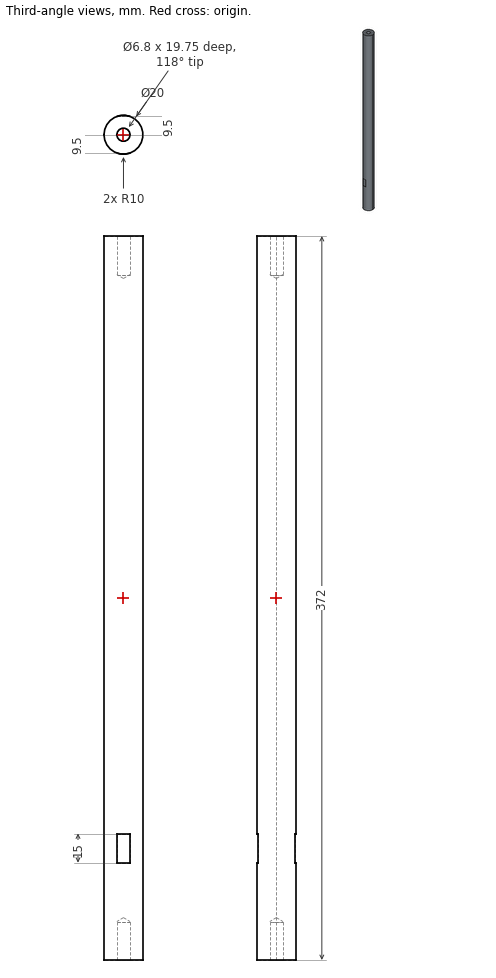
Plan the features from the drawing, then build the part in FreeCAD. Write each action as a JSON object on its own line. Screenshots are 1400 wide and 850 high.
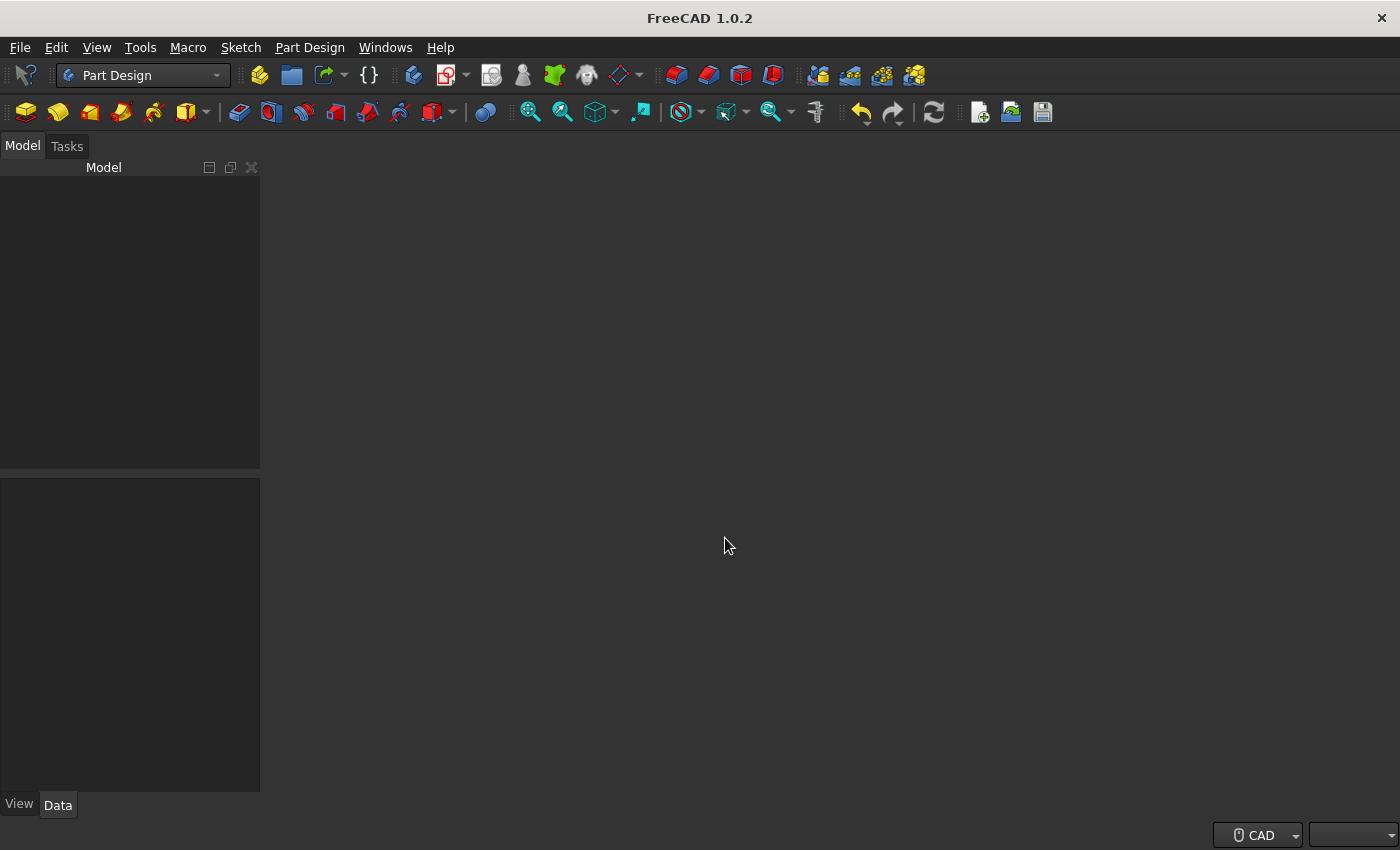
{"action": "left_click", "coordinate": [980, 112]}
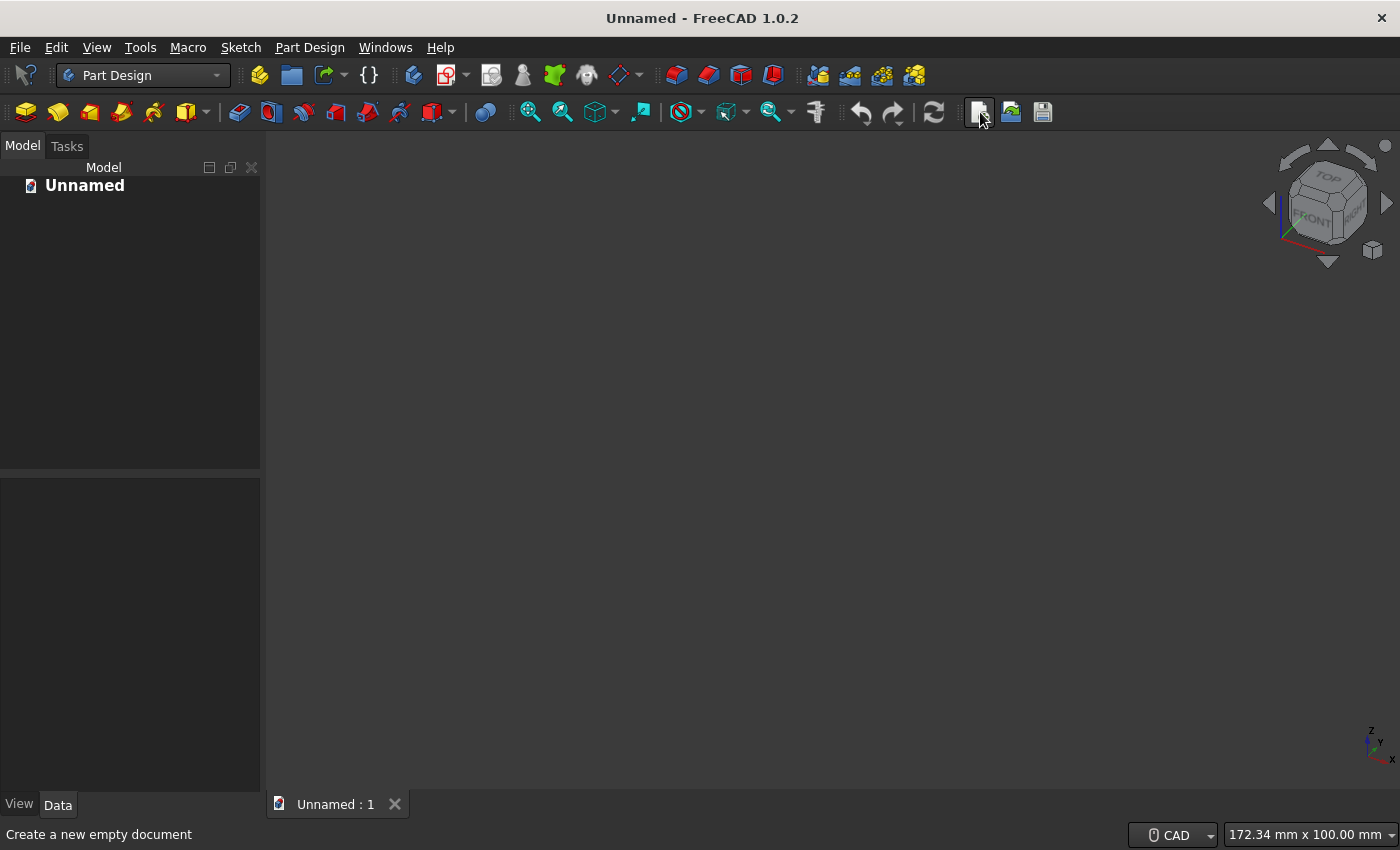
{"action": "left_click", "coordinate": [446, 76]}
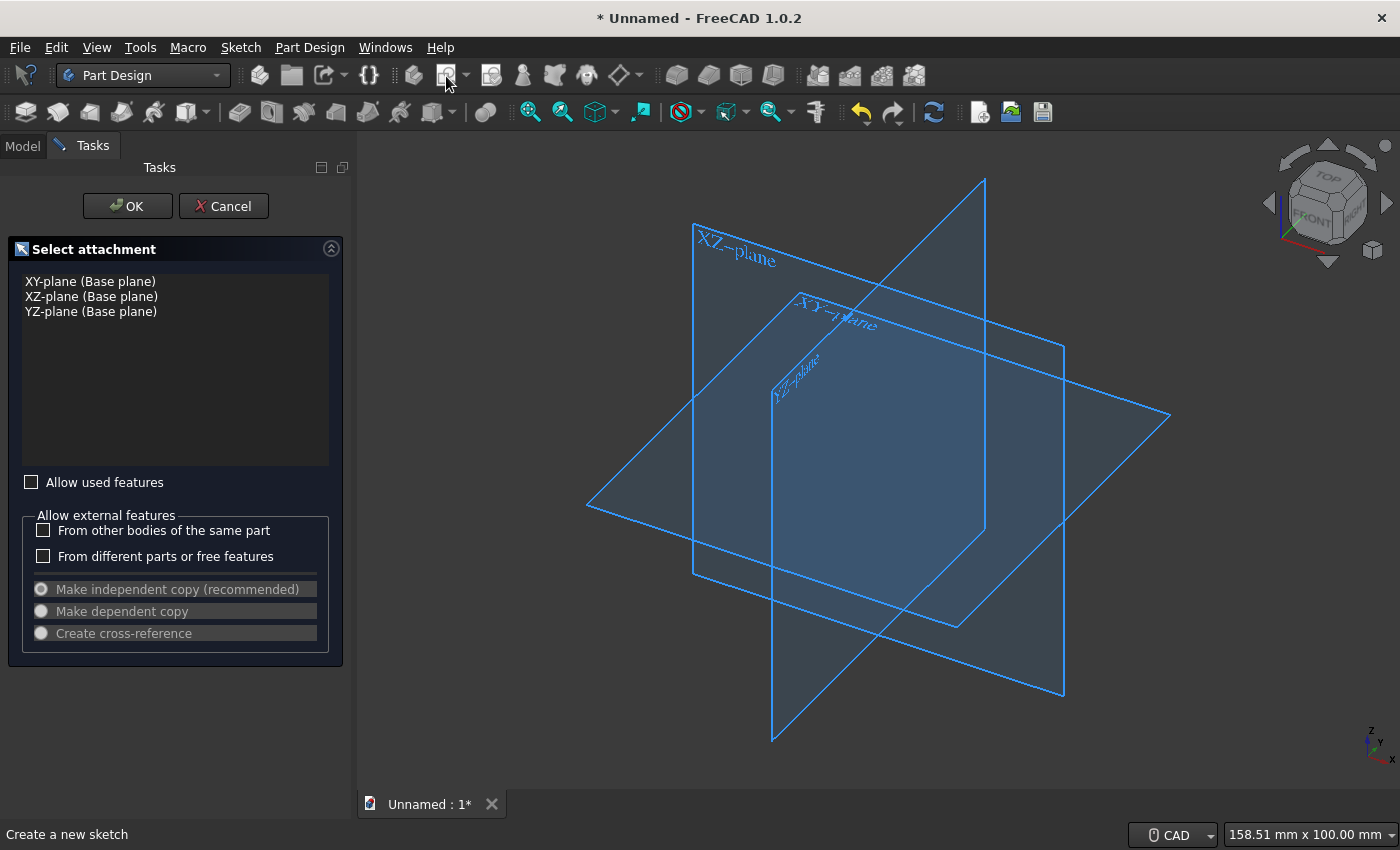
{"action": "left_click", "coordinate": [82, 282]}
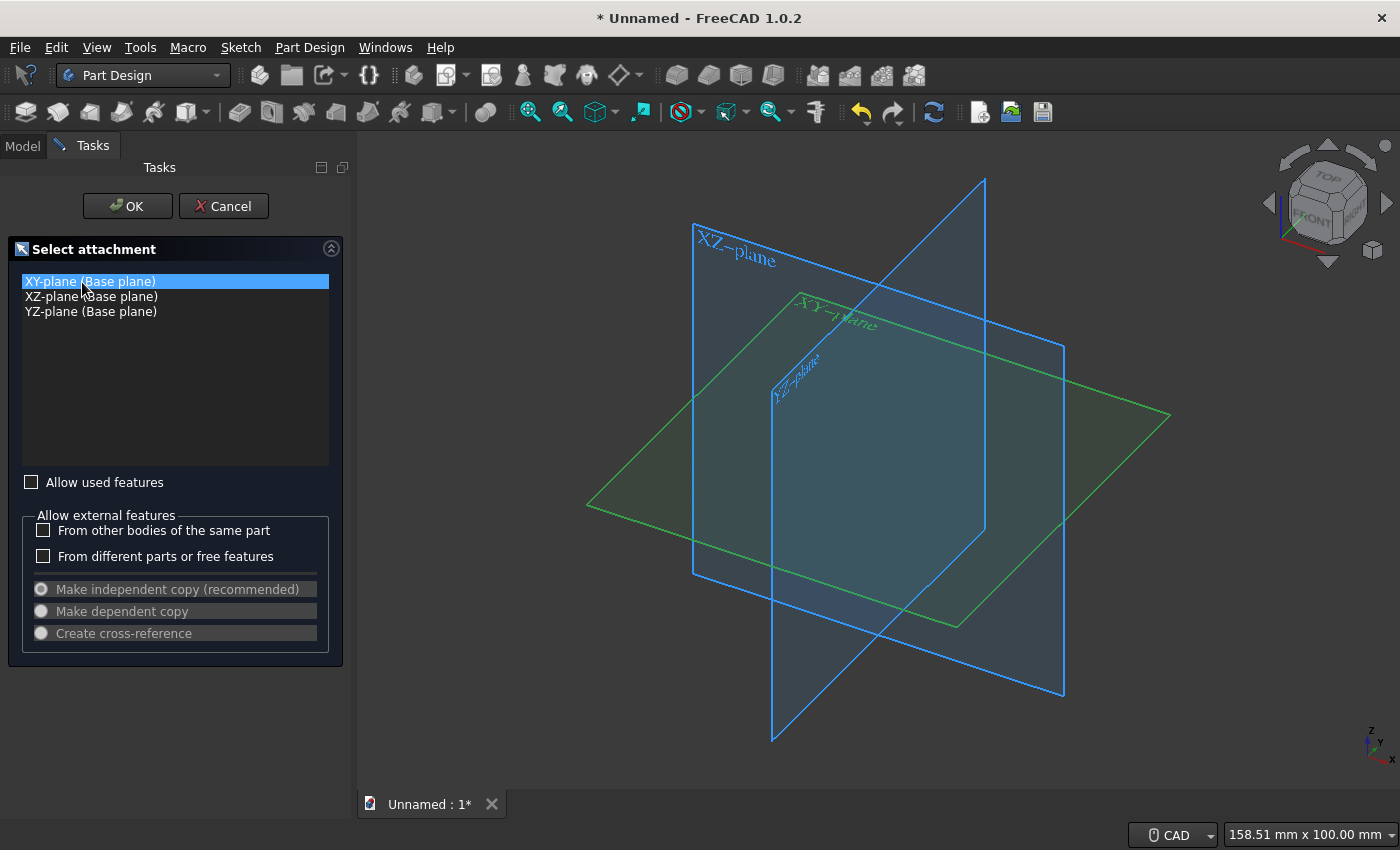
{"action": "left_click", "coordinate": [128, 206]}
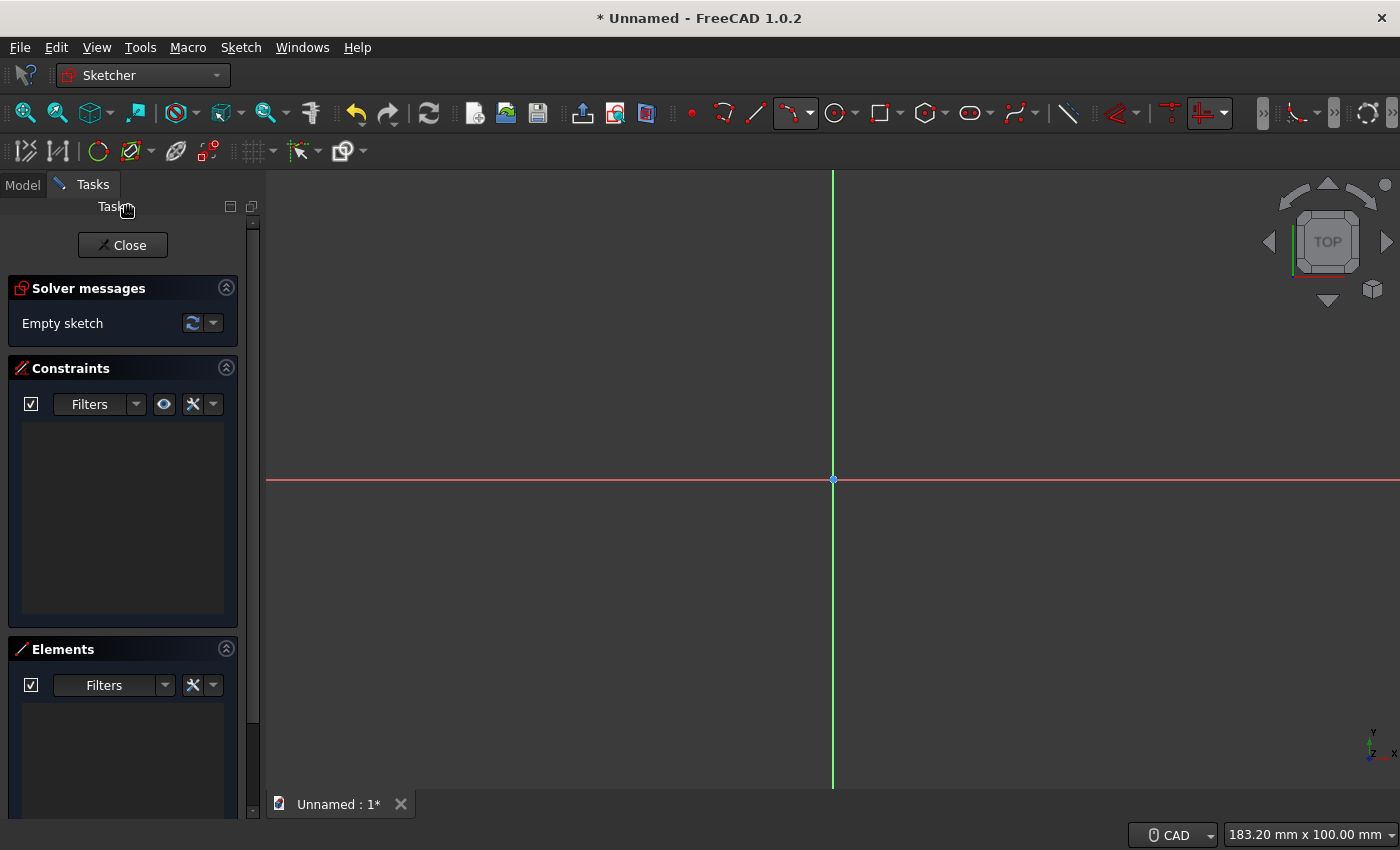
{"action": "scroll", "coordinate": [863, 480], "scroll_direction": "up", "scroll_amount": 6}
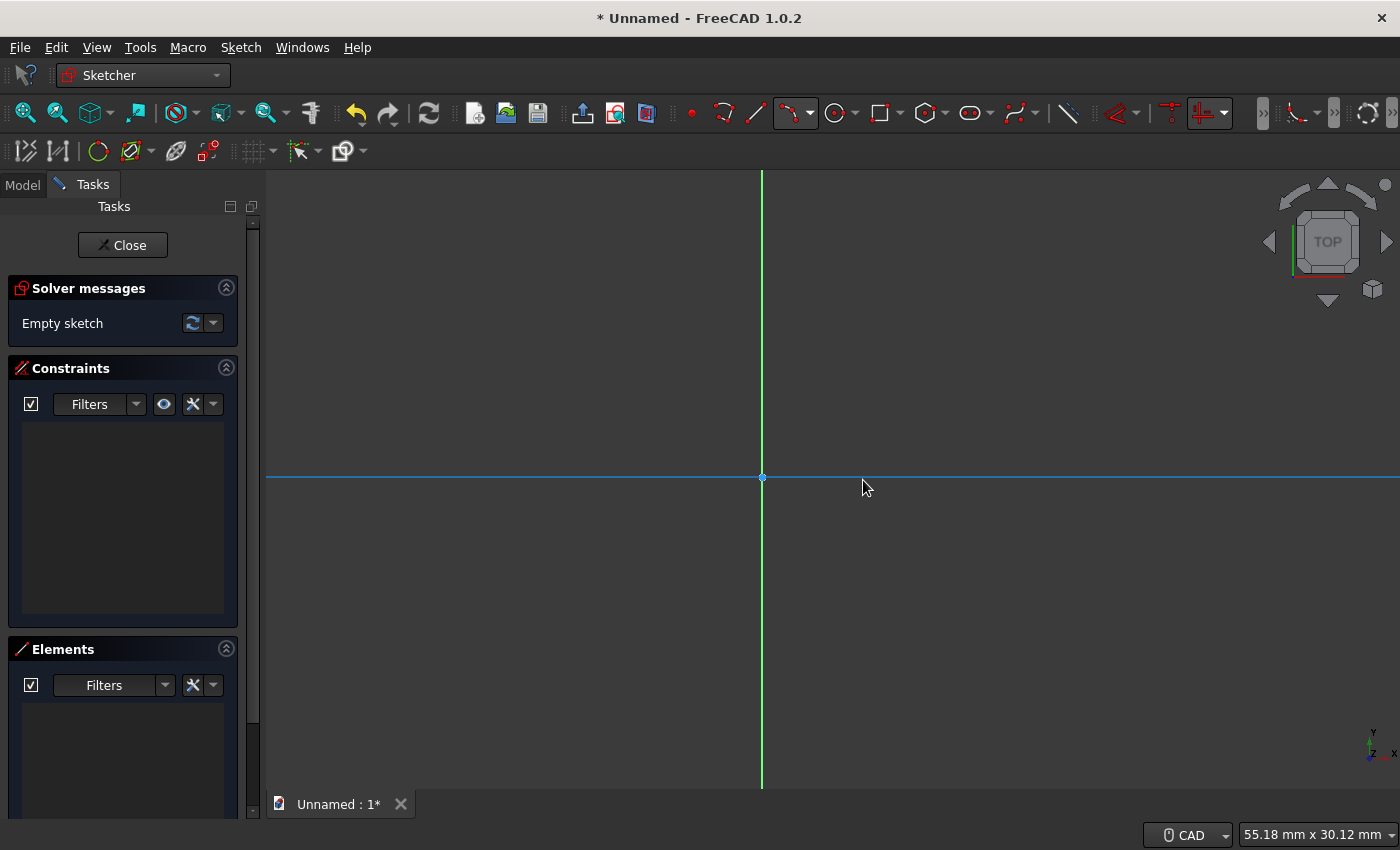
{"action": "left_click", "coordinate": [836, 114]}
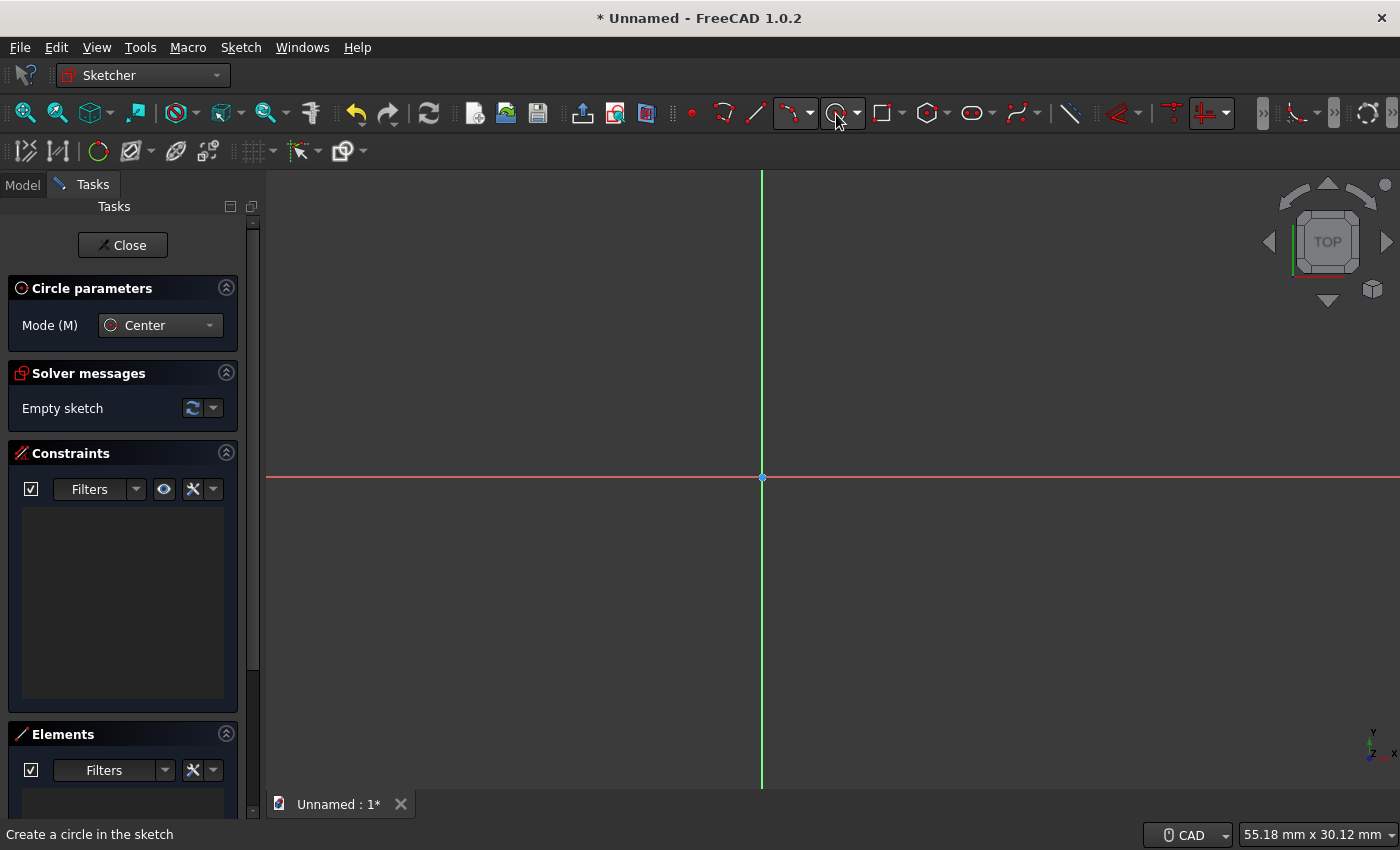
{"action": "left_click", "coordinate": [762, 477]}
{"action": "left_click", "coordinate": [907, 332]}
{"action": "key", "text": "Escape"}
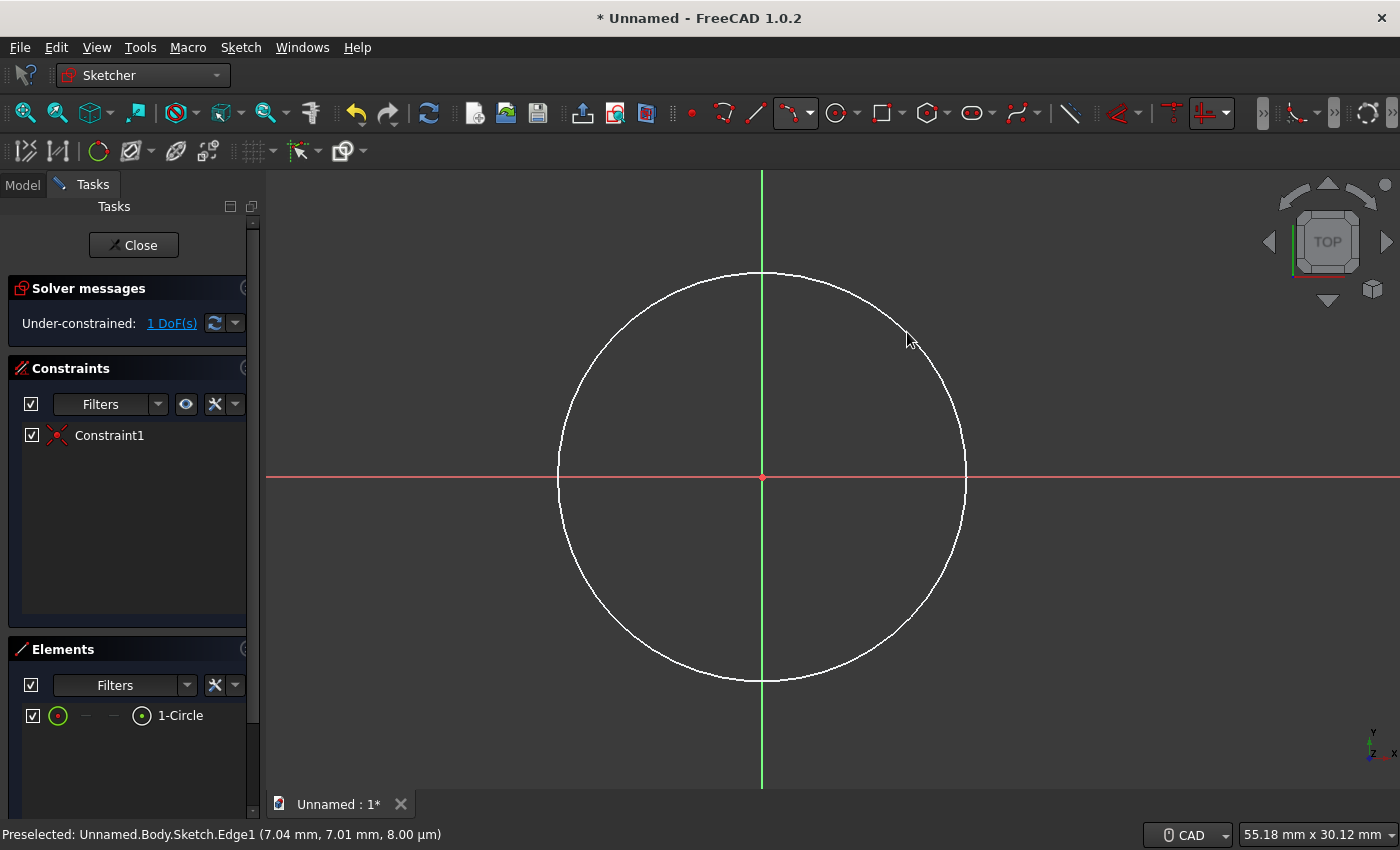
{"action": "left_click", "coordinate": [906, 332]}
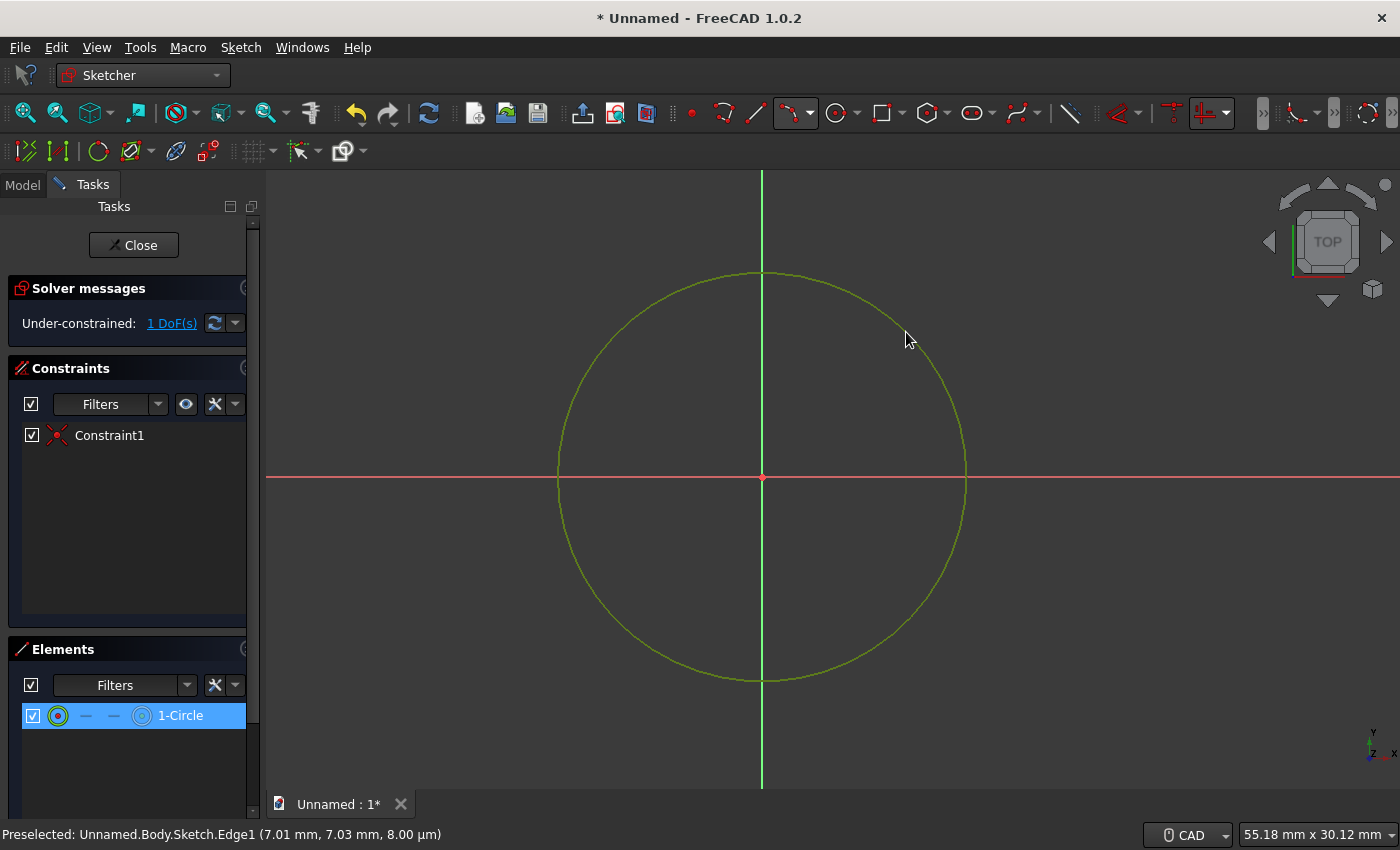
{"action": "left_click", "coordinate": [1140, 114]}